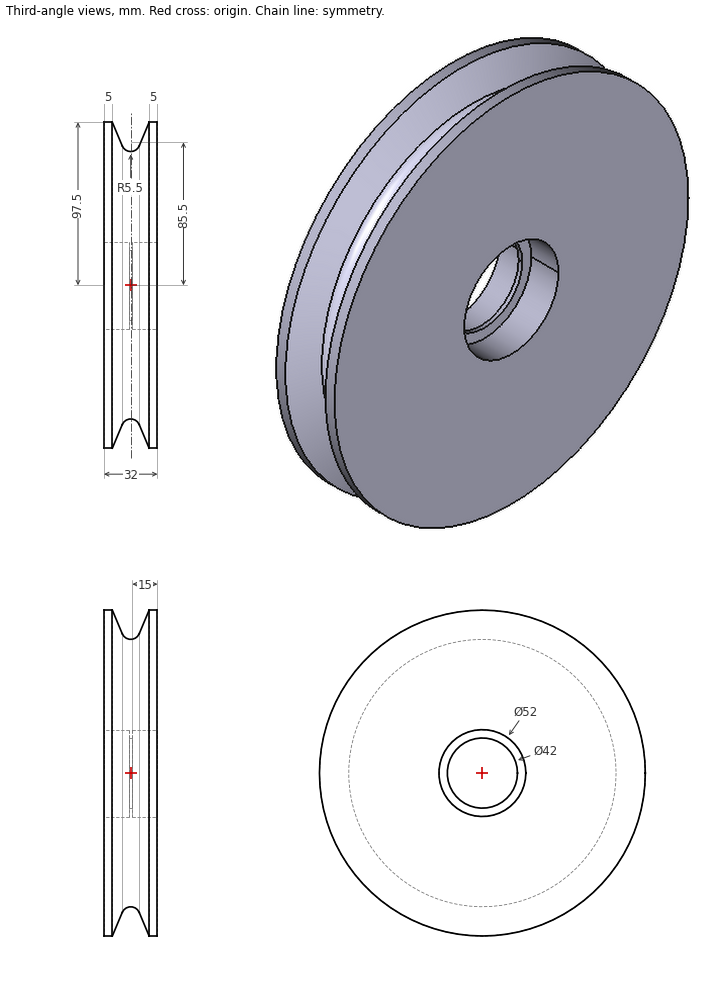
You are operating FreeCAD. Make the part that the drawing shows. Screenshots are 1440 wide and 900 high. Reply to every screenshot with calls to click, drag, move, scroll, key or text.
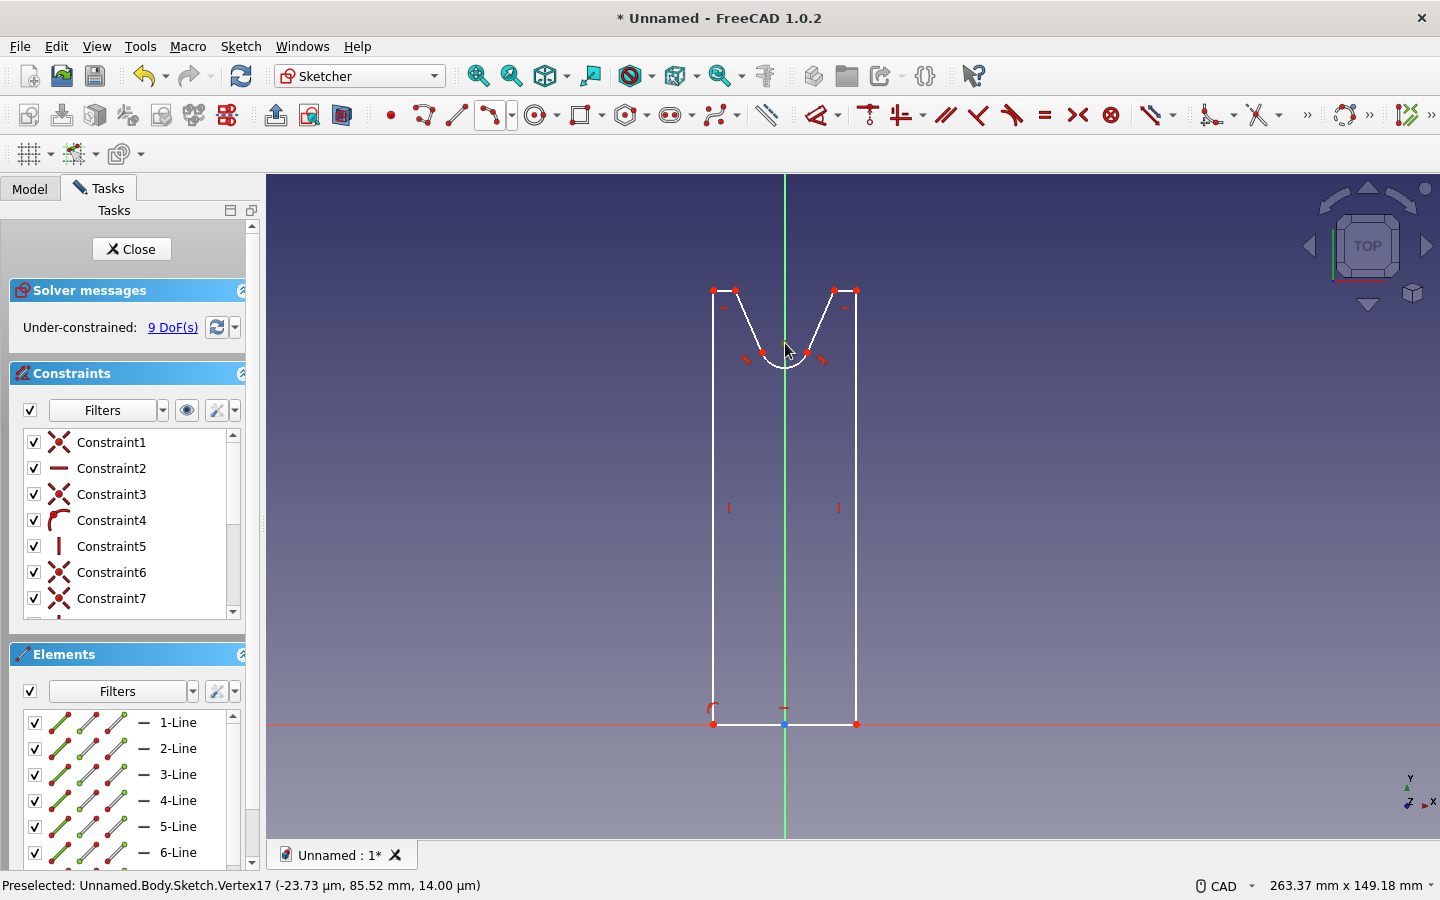
click(785, 768)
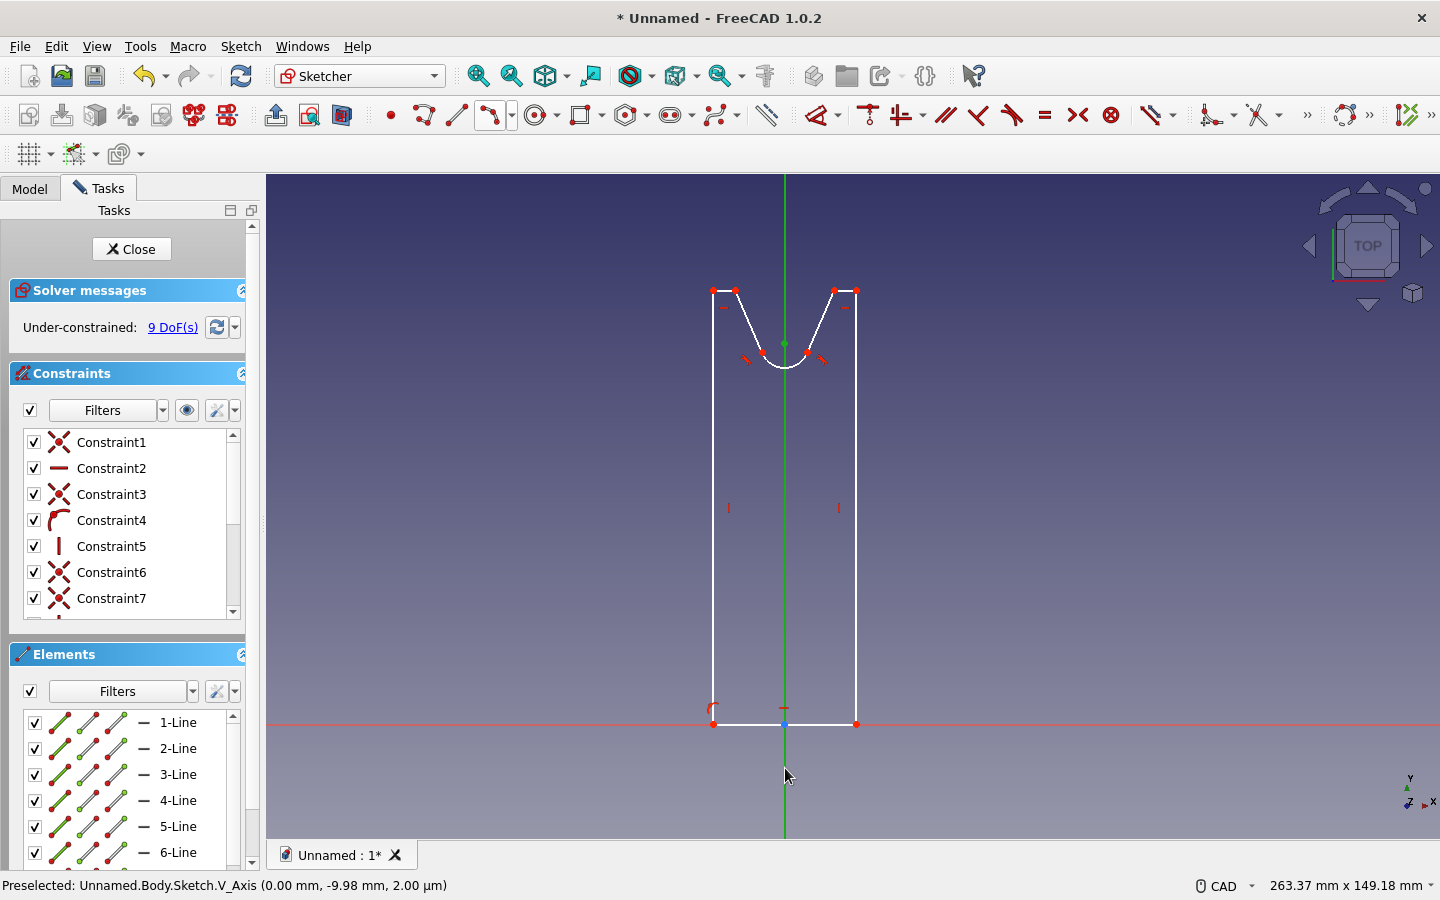
click(868, 116)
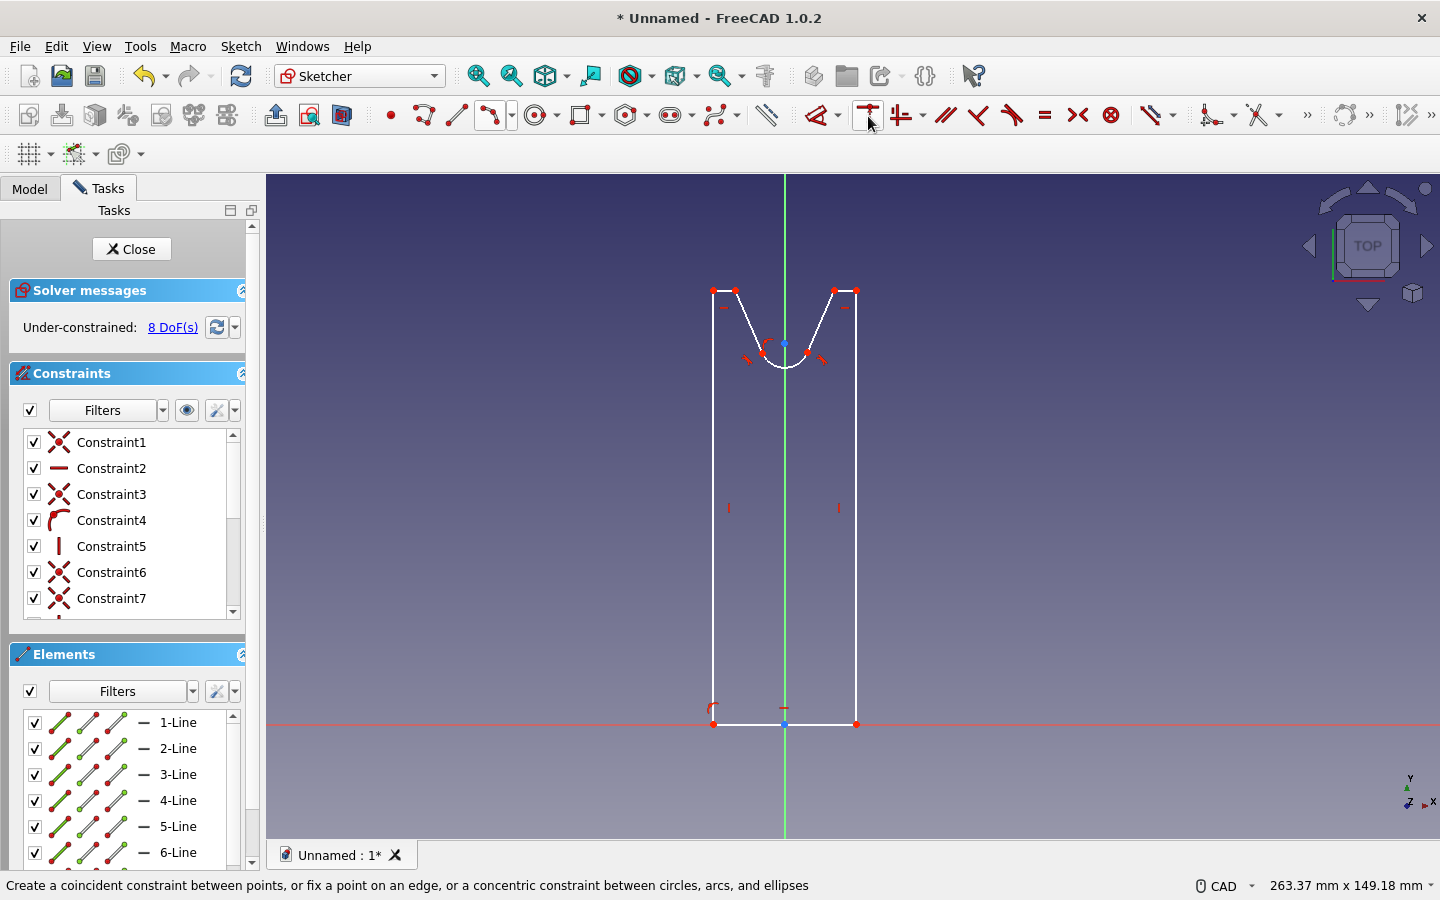
click(713, 291)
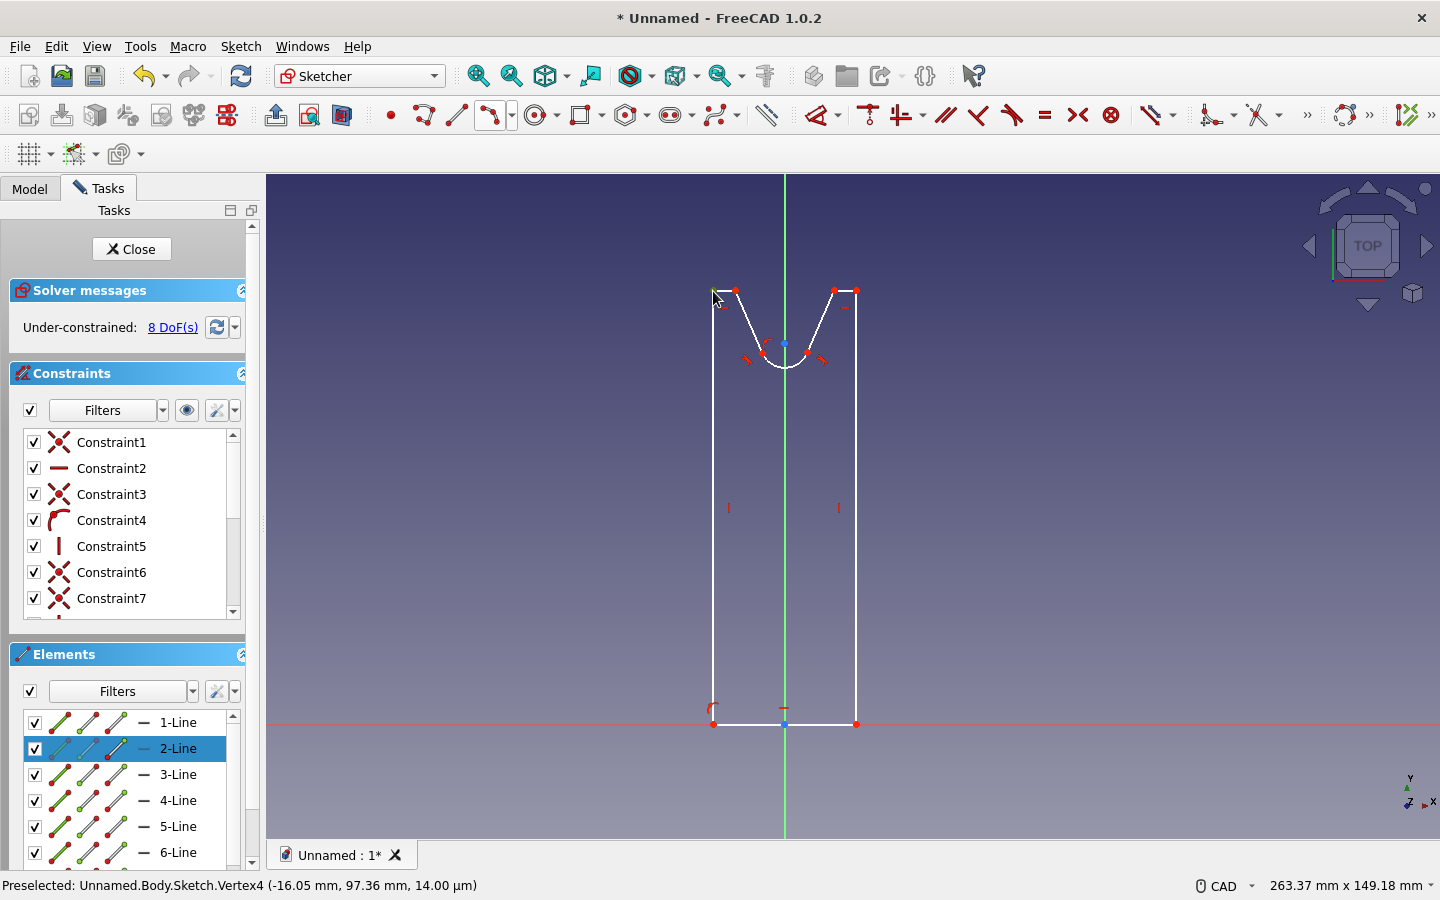
click(856, 291)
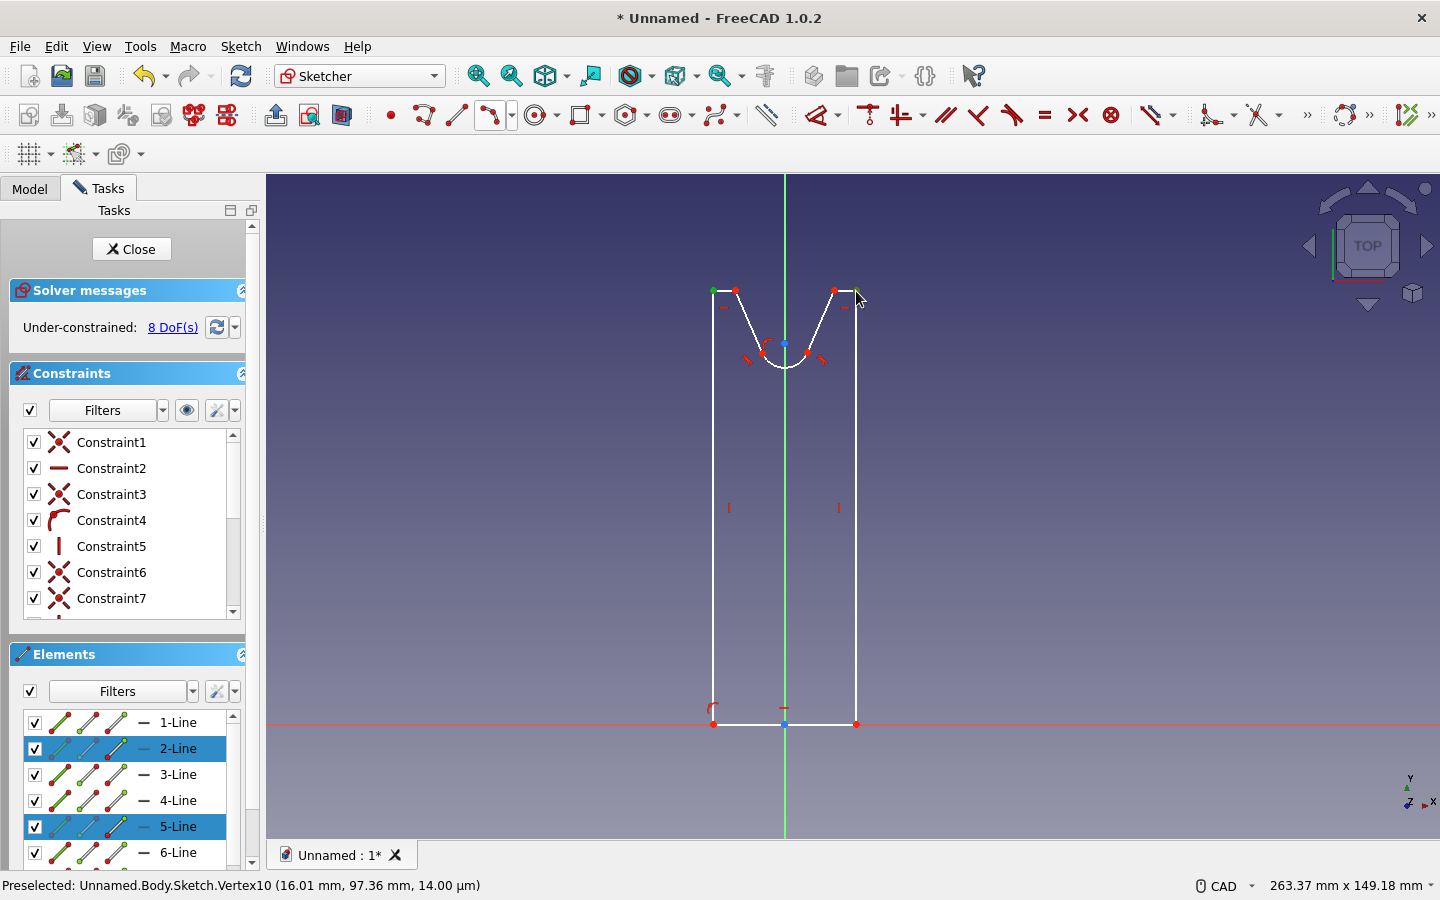
click(785, 768)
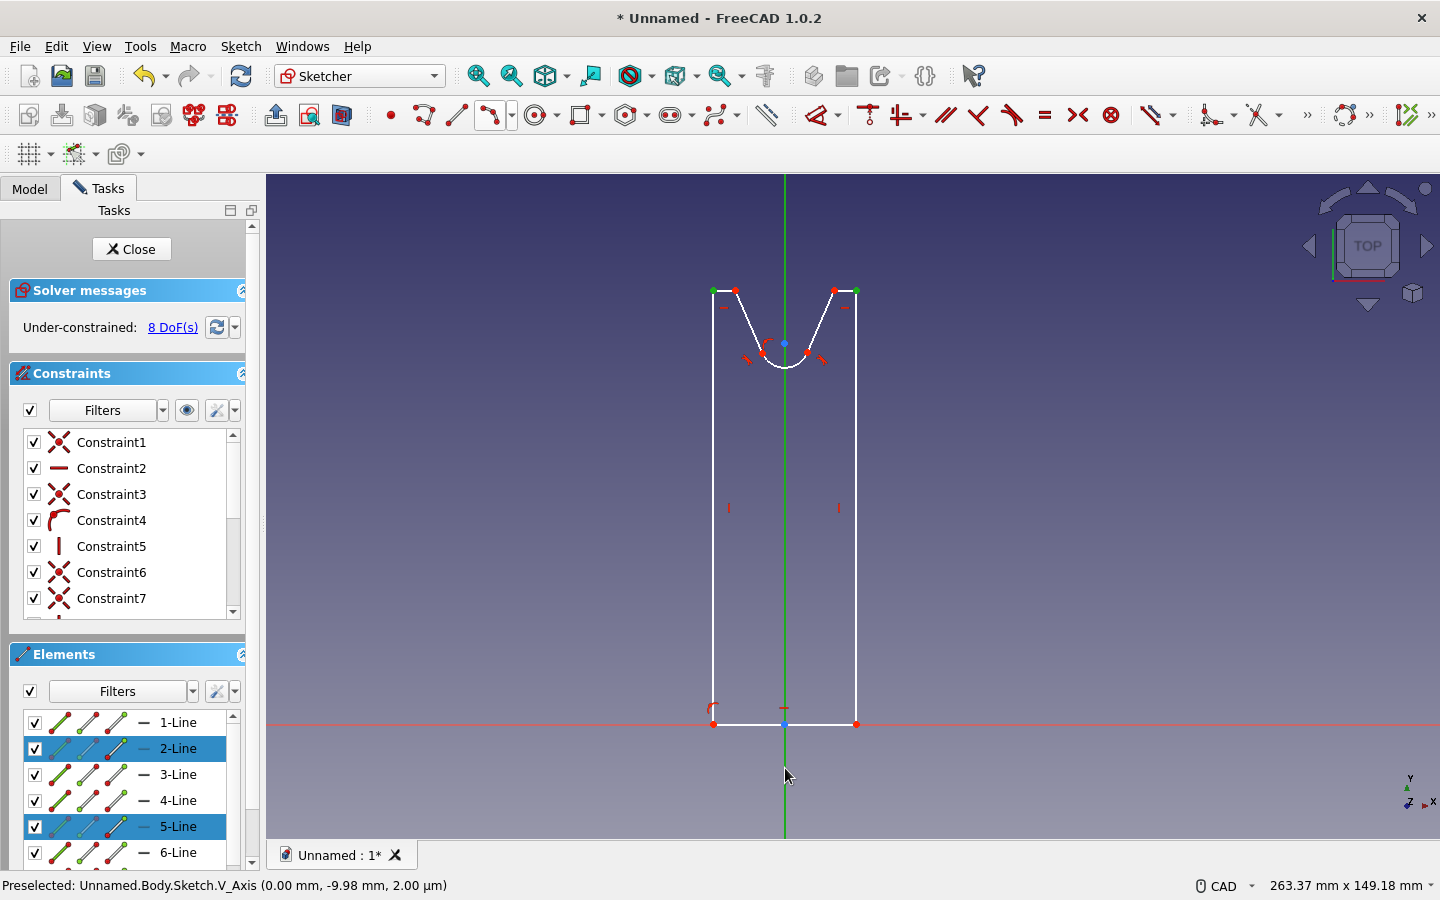
click(1078, 116)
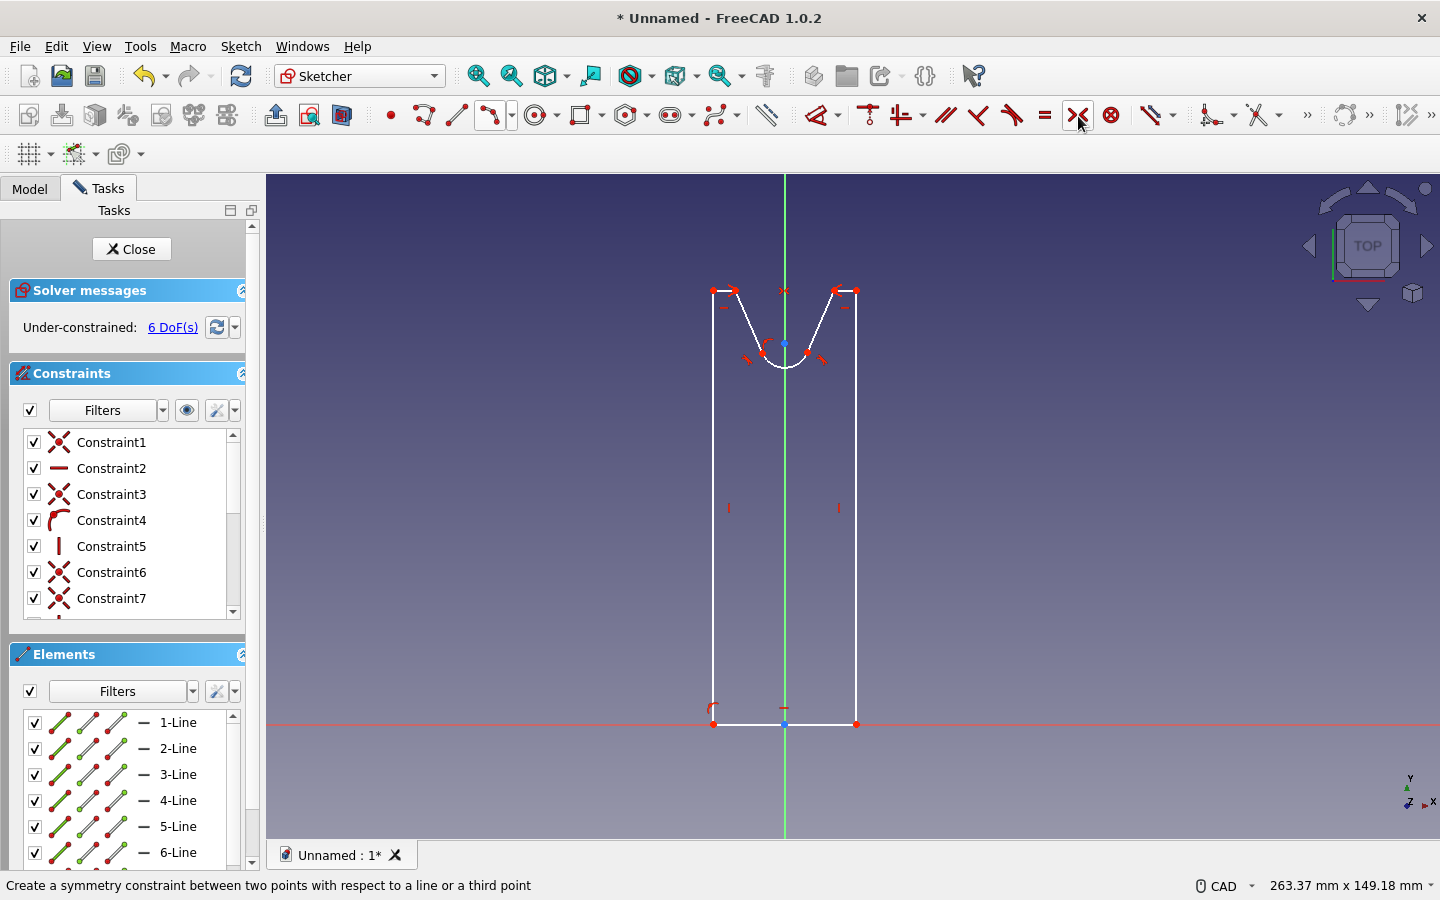
click(816, 116)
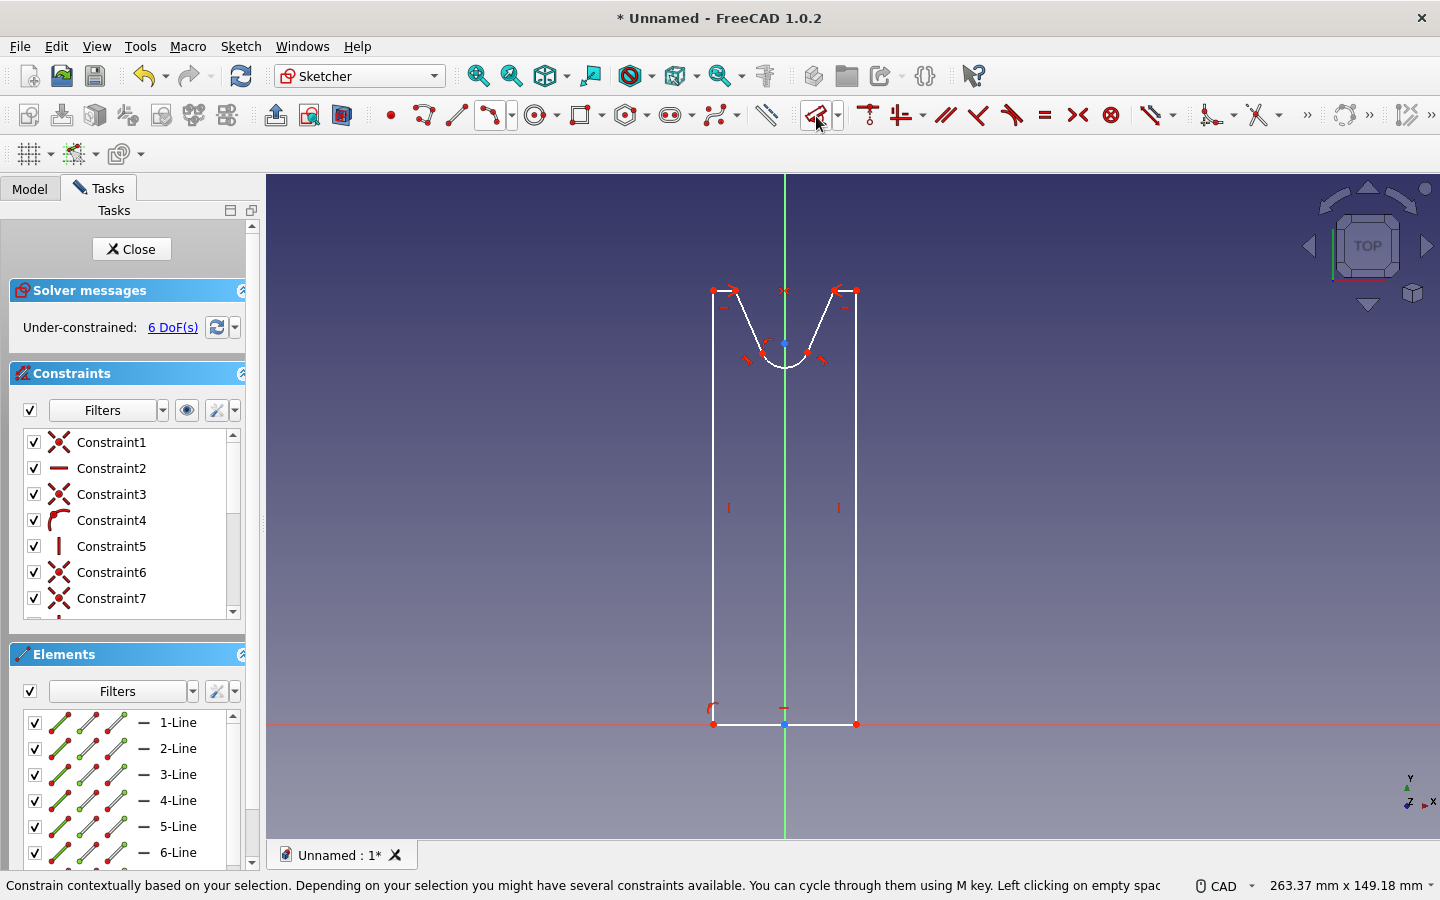
scroll(774, 365, up, 3)